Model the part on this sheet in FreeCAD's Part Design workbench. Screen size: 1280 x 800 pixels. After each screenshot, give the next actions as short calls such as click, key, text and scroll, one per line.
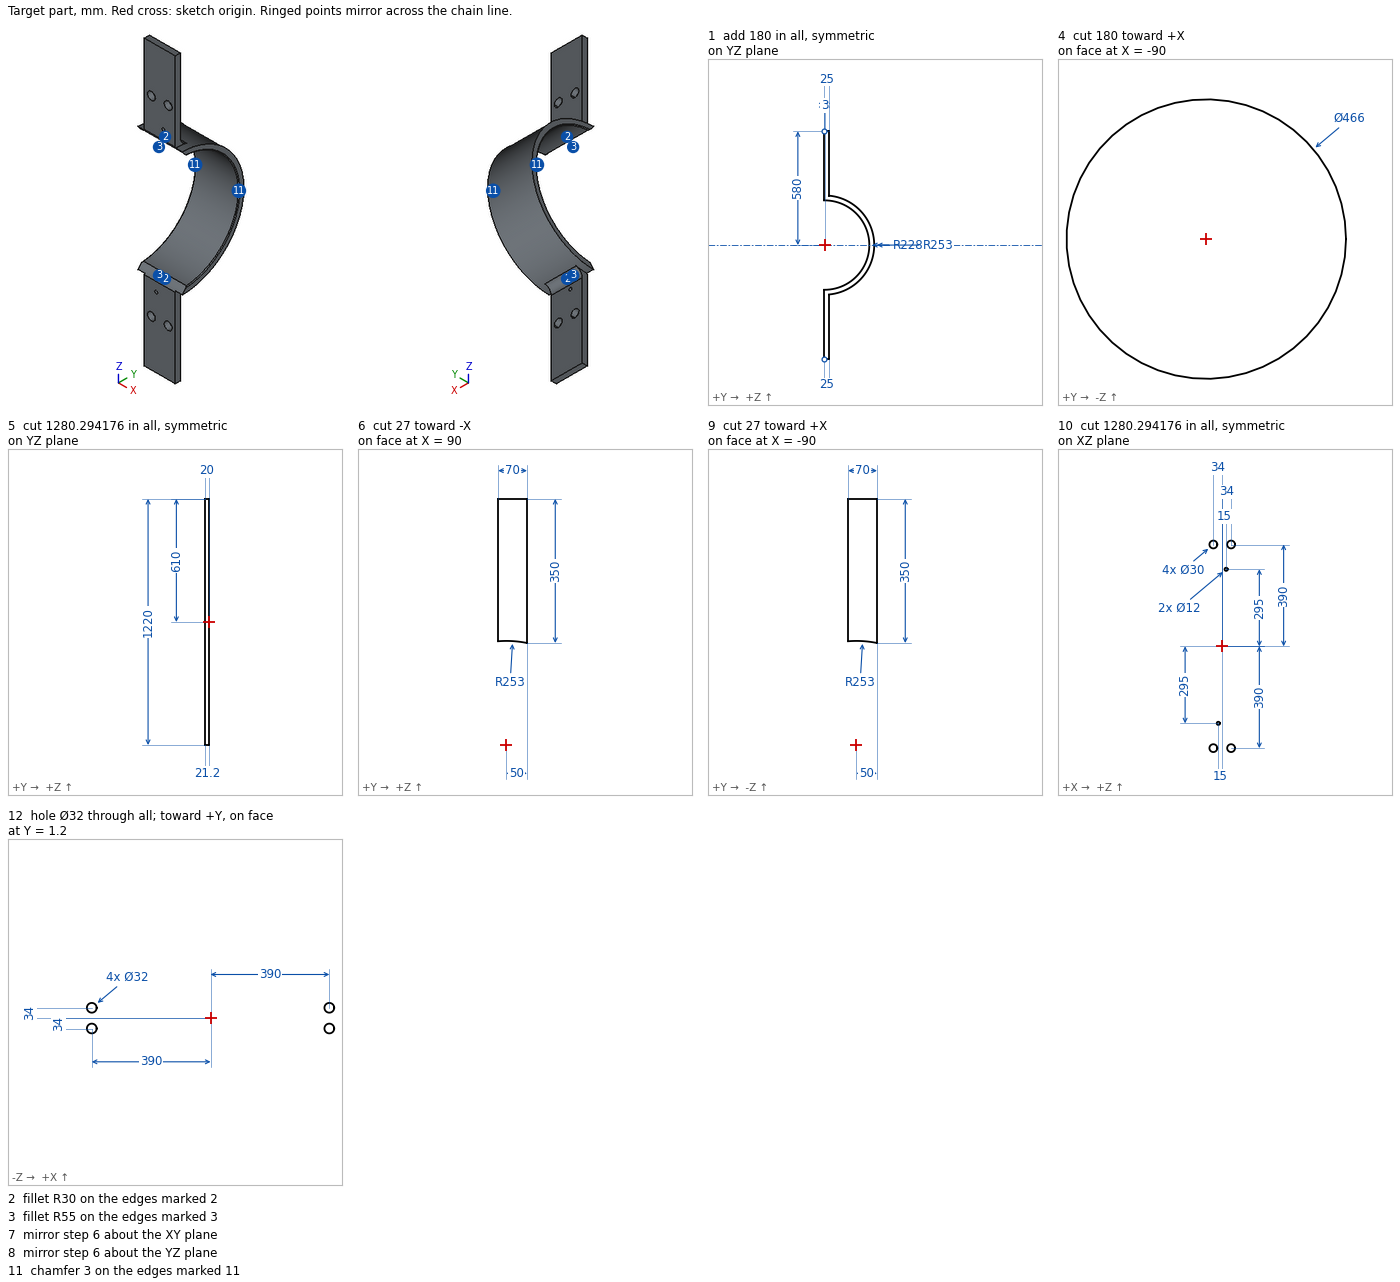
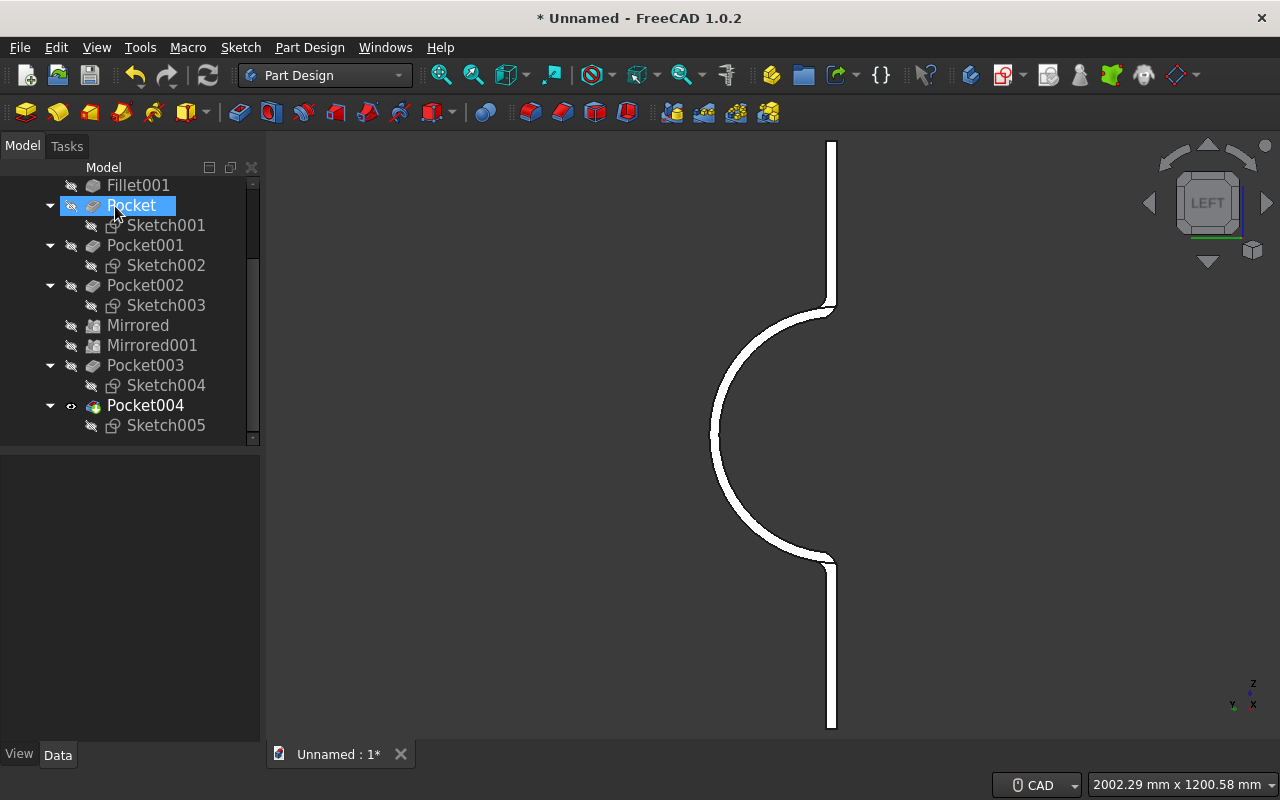
click(750, 513)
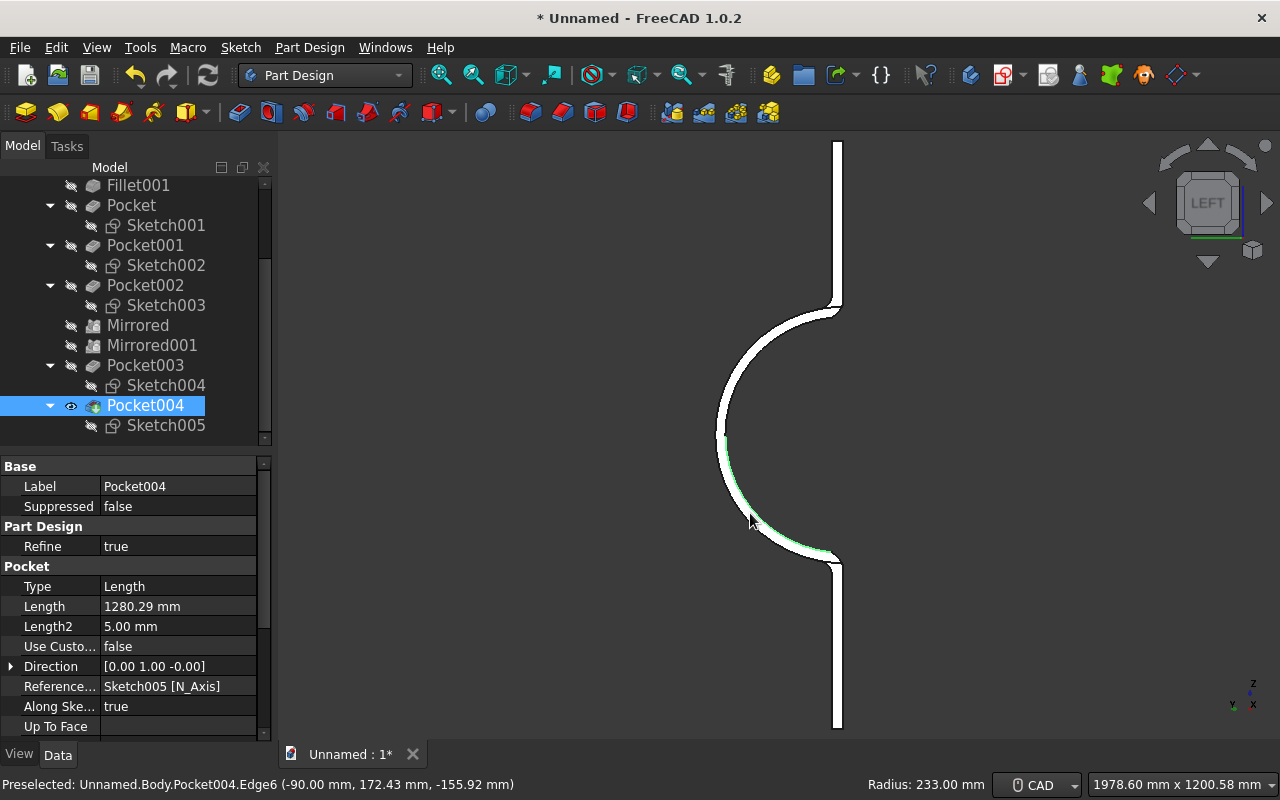
key(0)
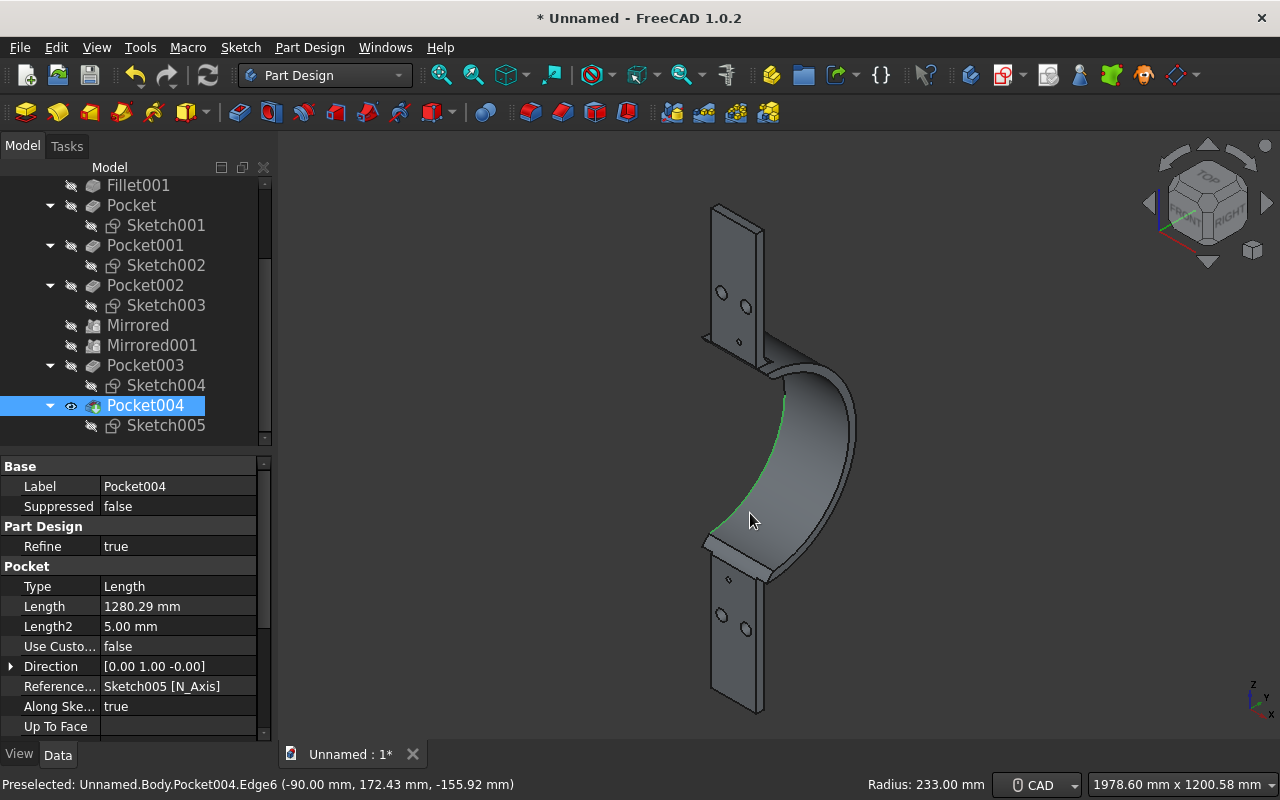
click(827, 378, ctrl)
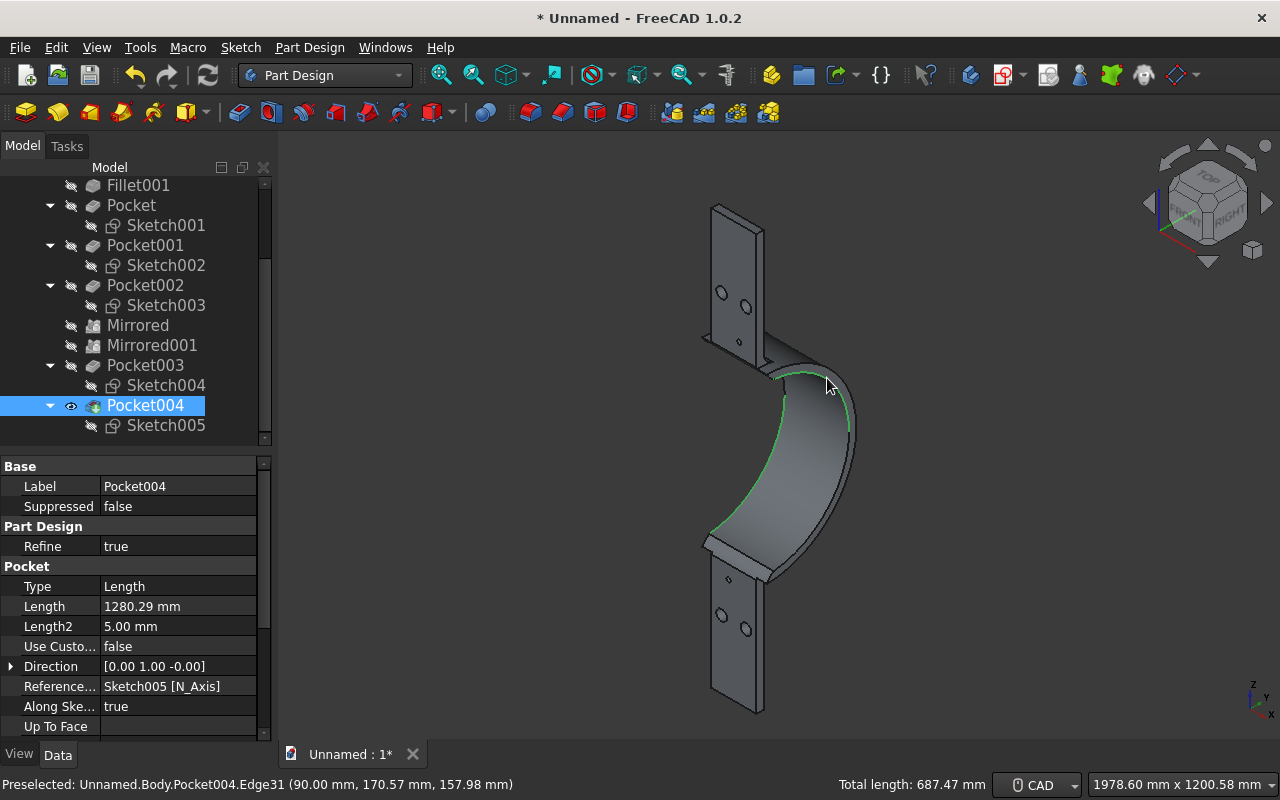
click(564, 112)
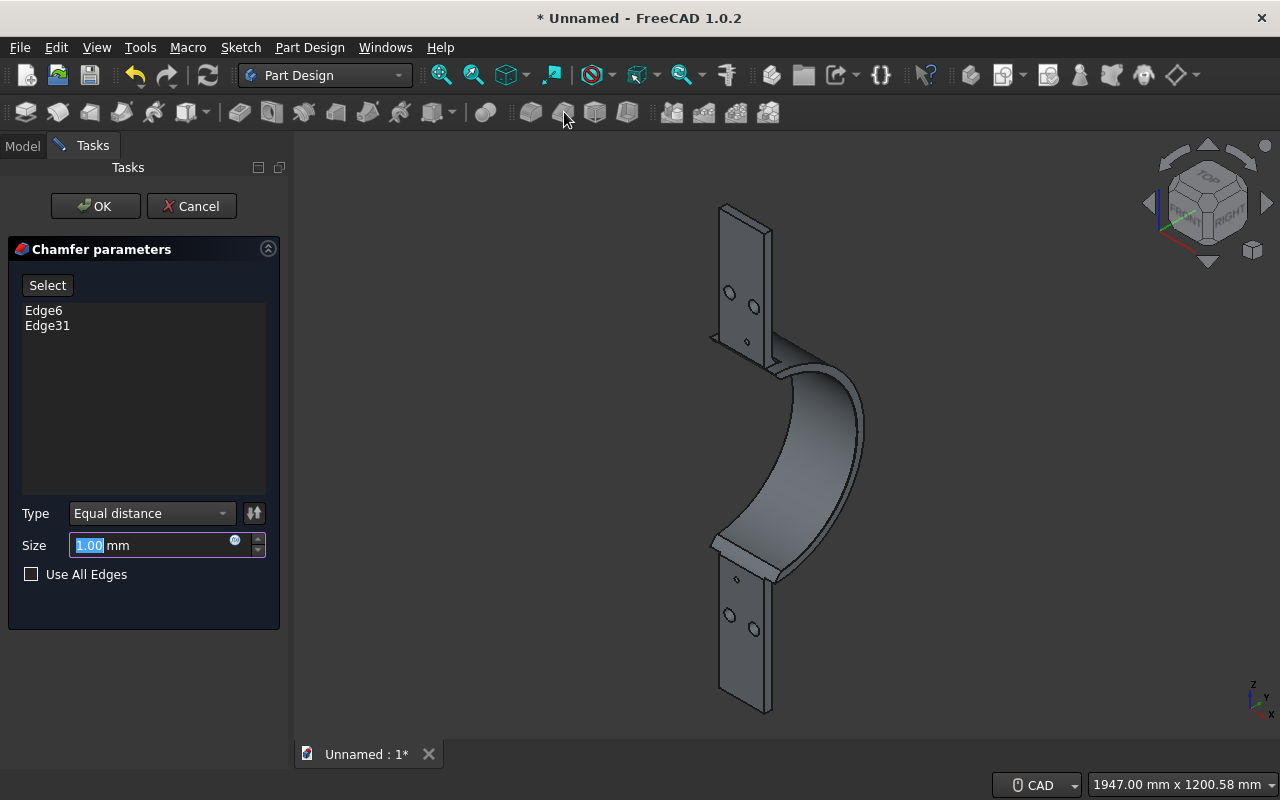
text(3)
key(Tab)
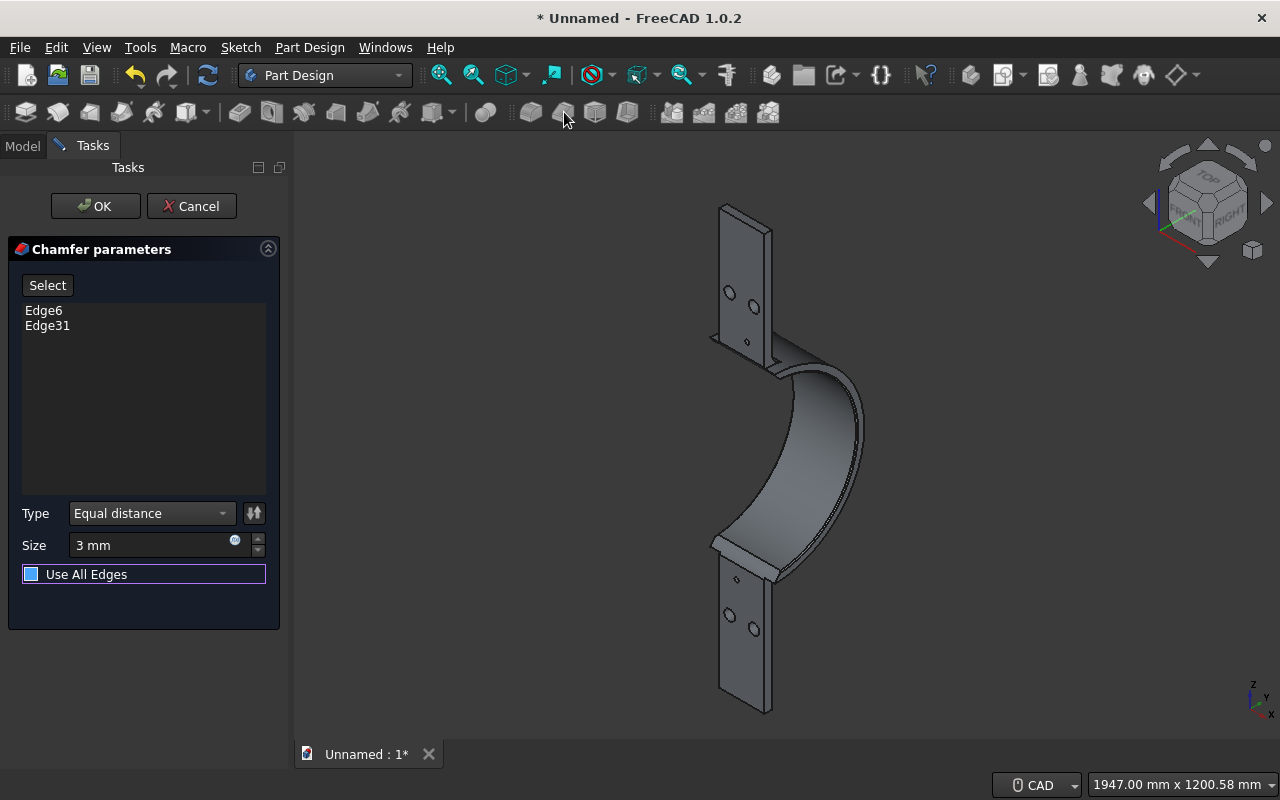
click(96, 206)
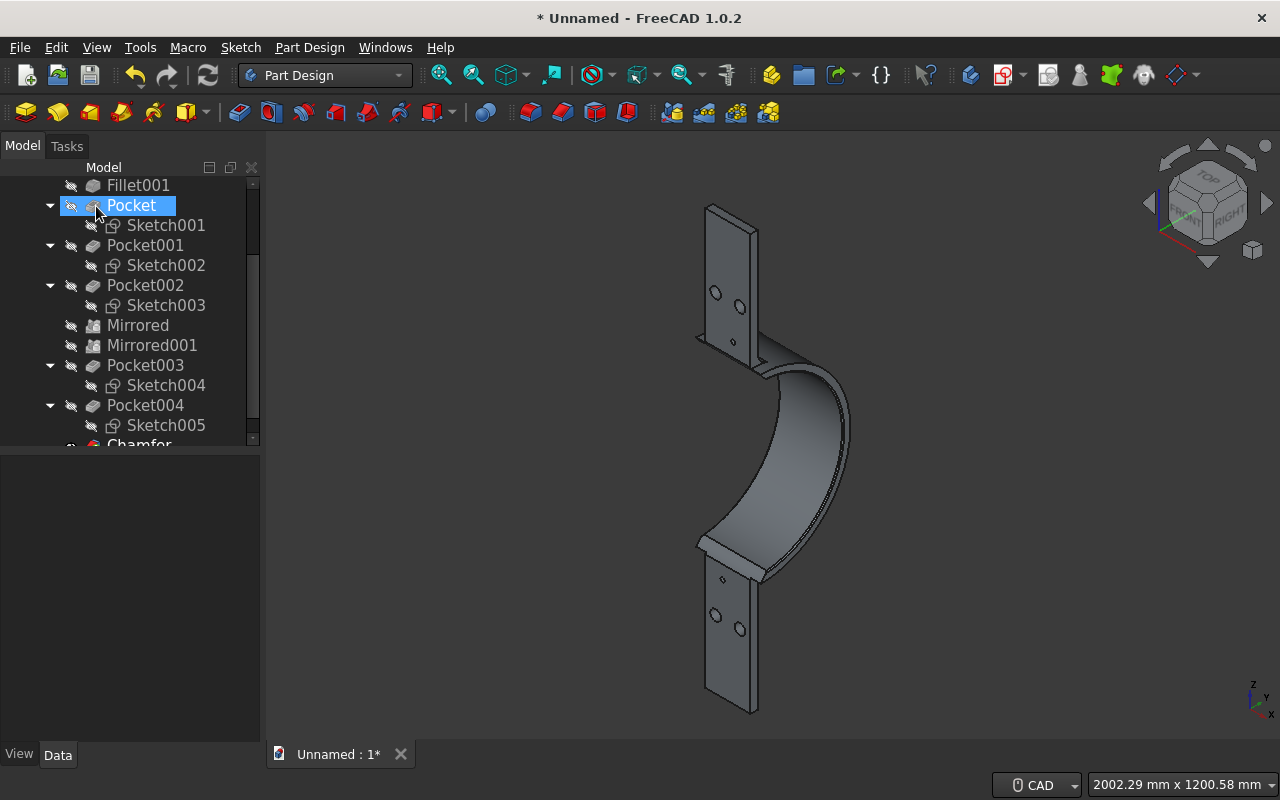
click(728, 671)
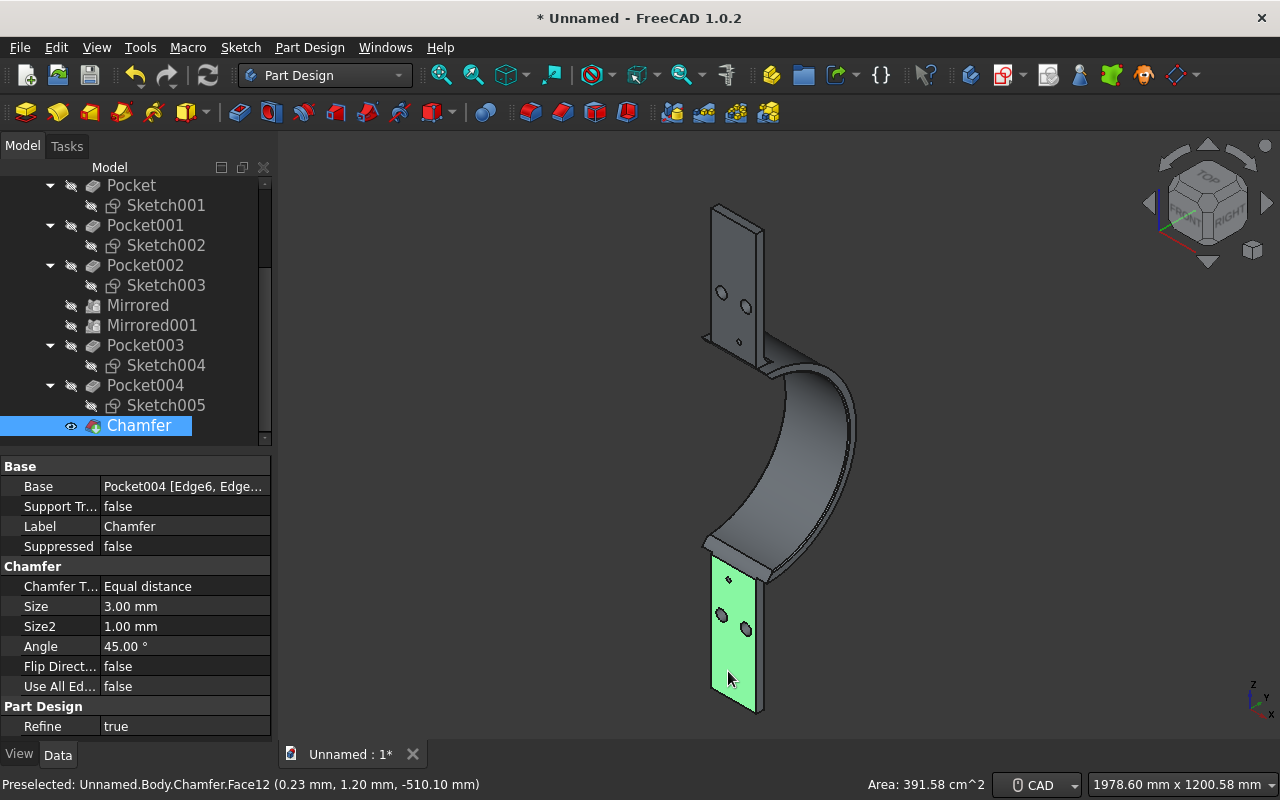
click(1004, 76)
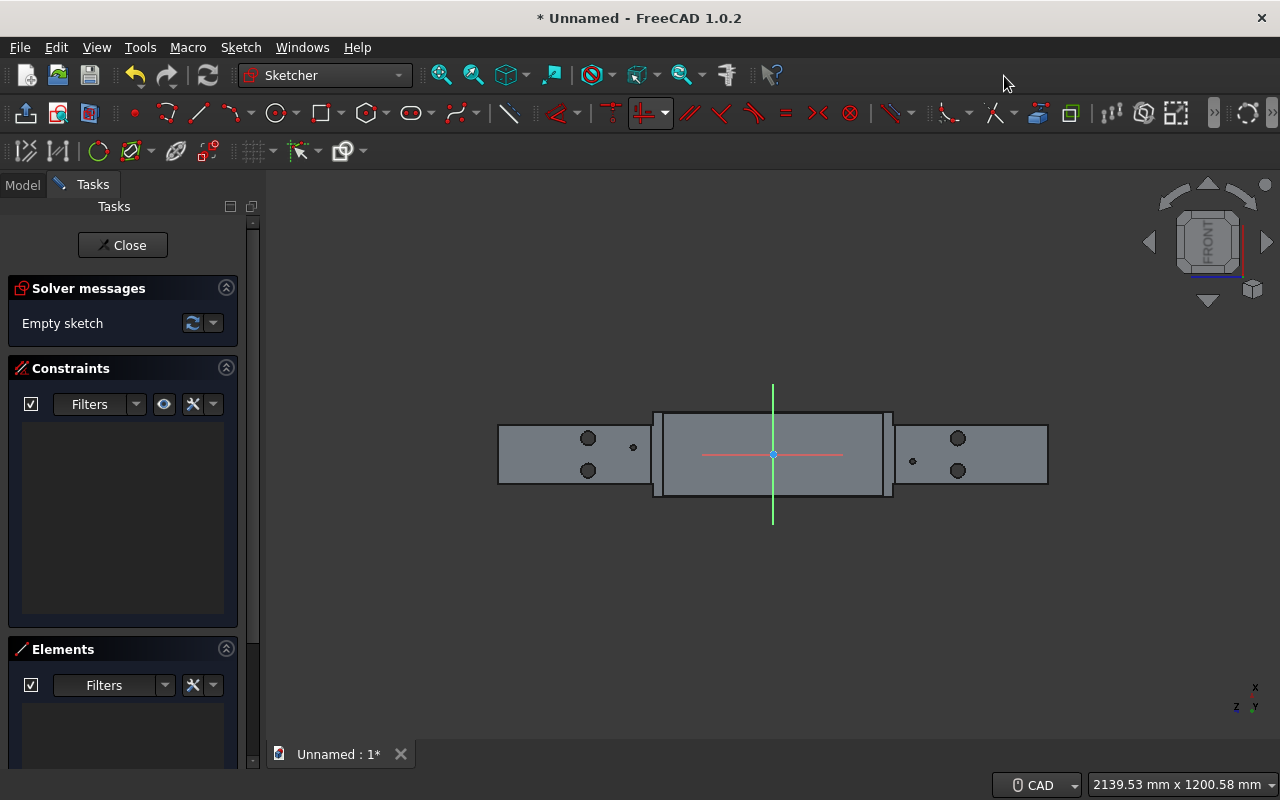
scroll(912, 454, up, 2)